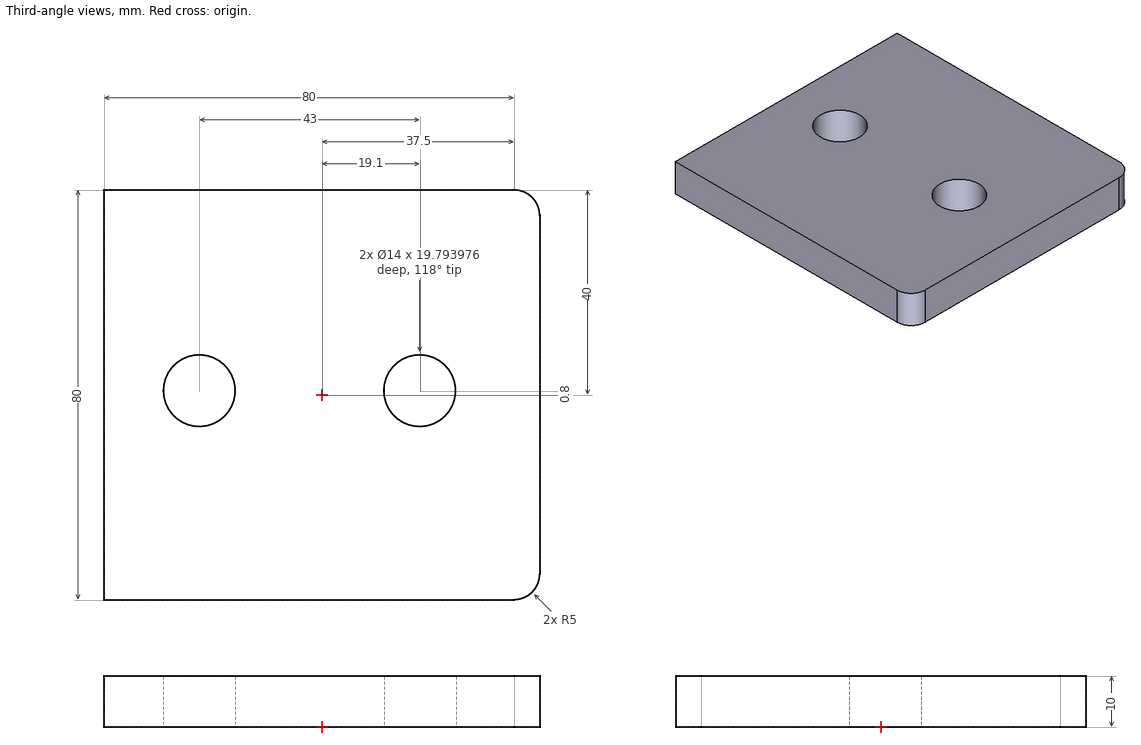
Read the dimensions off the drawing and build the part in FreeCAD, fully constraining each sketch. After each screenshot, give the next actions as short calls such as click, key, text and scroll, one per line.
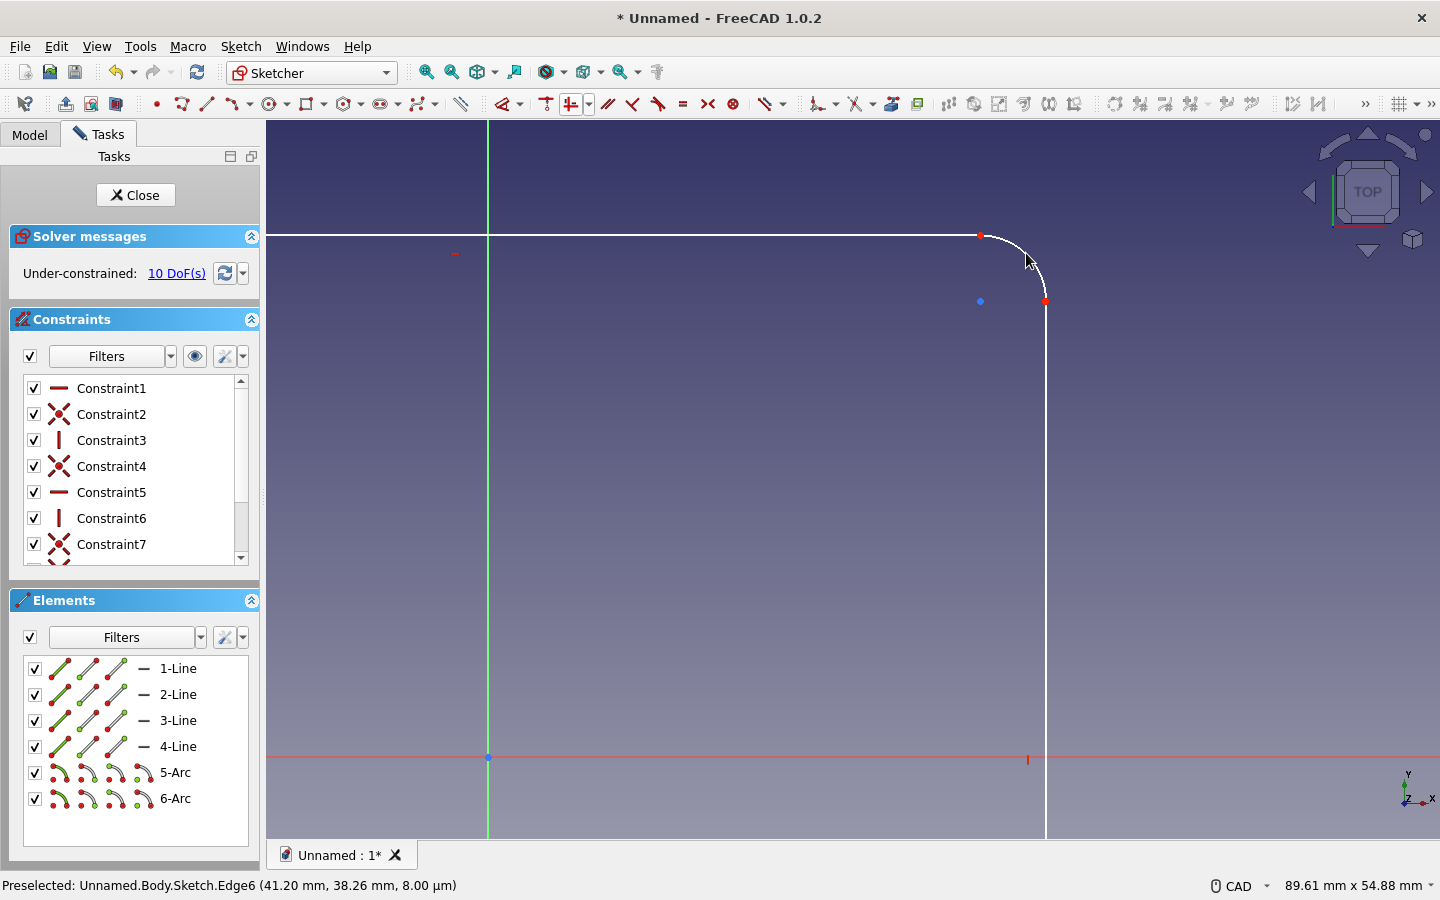
click(666, 235)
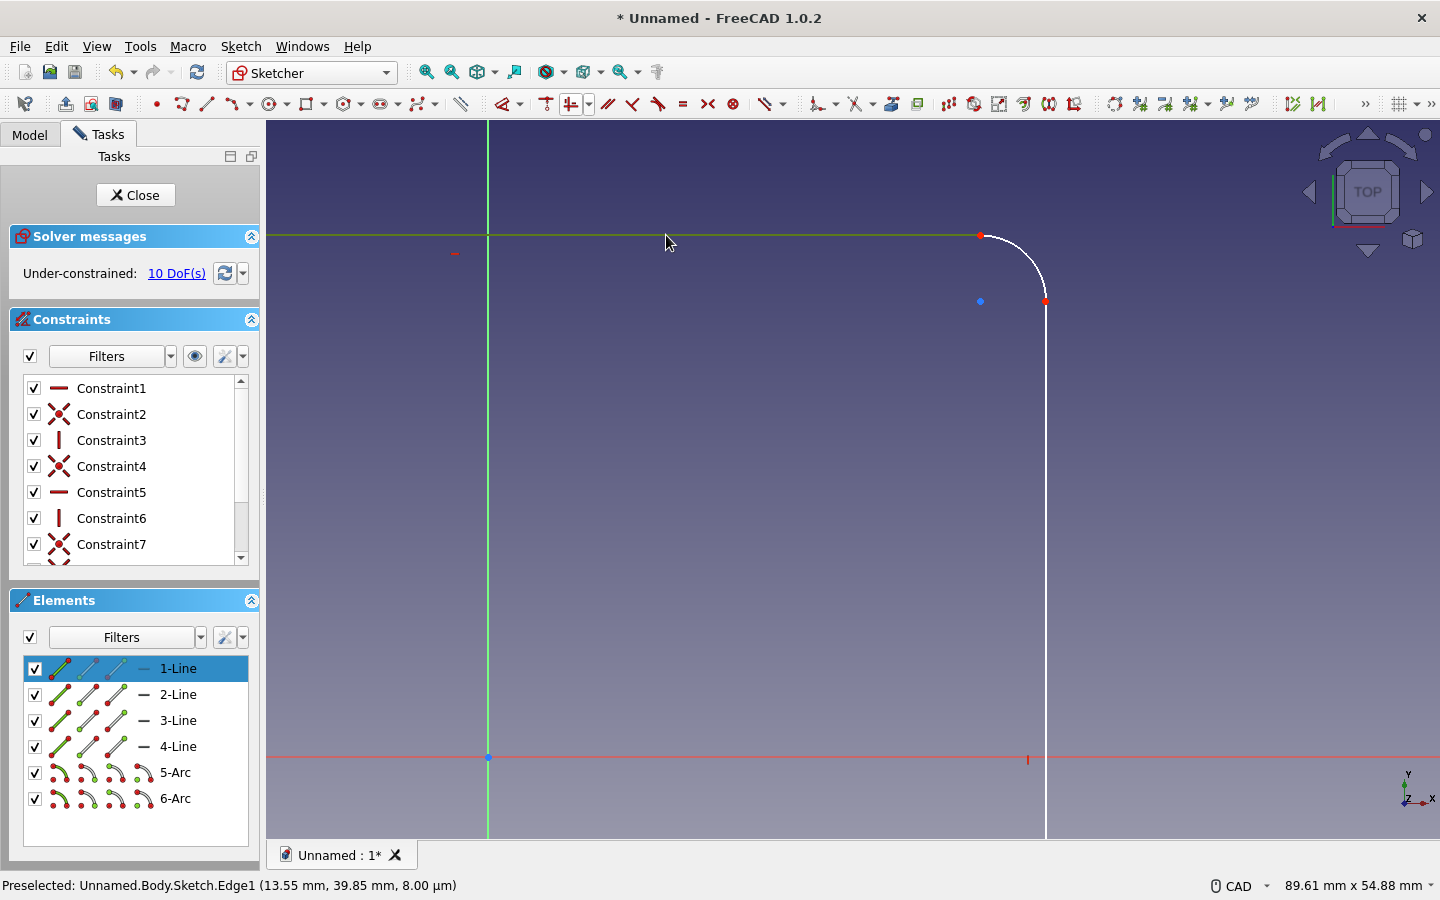
click(1039, 271)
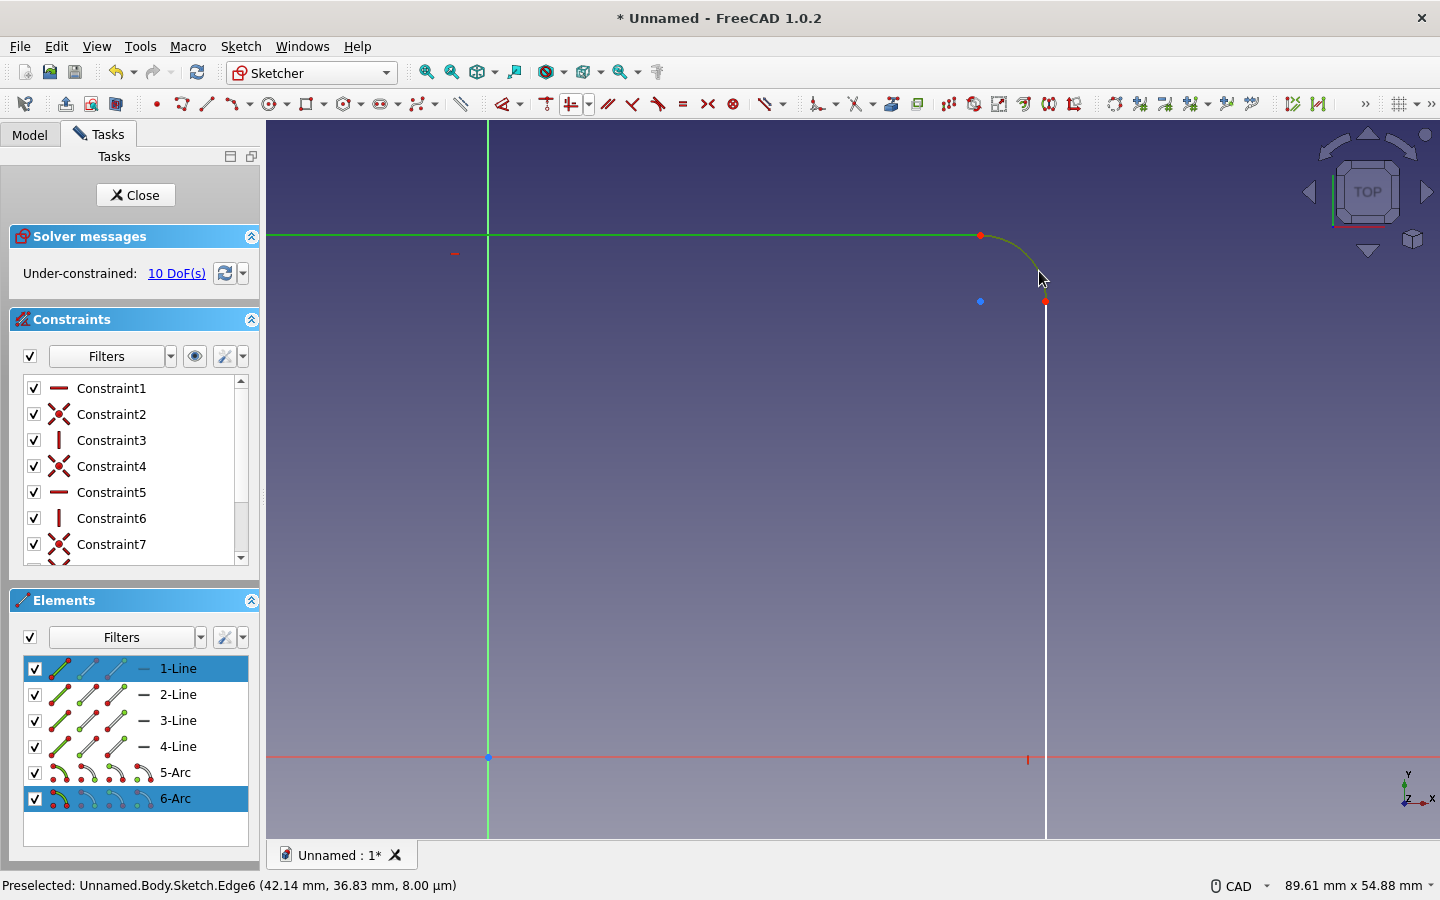
key(t)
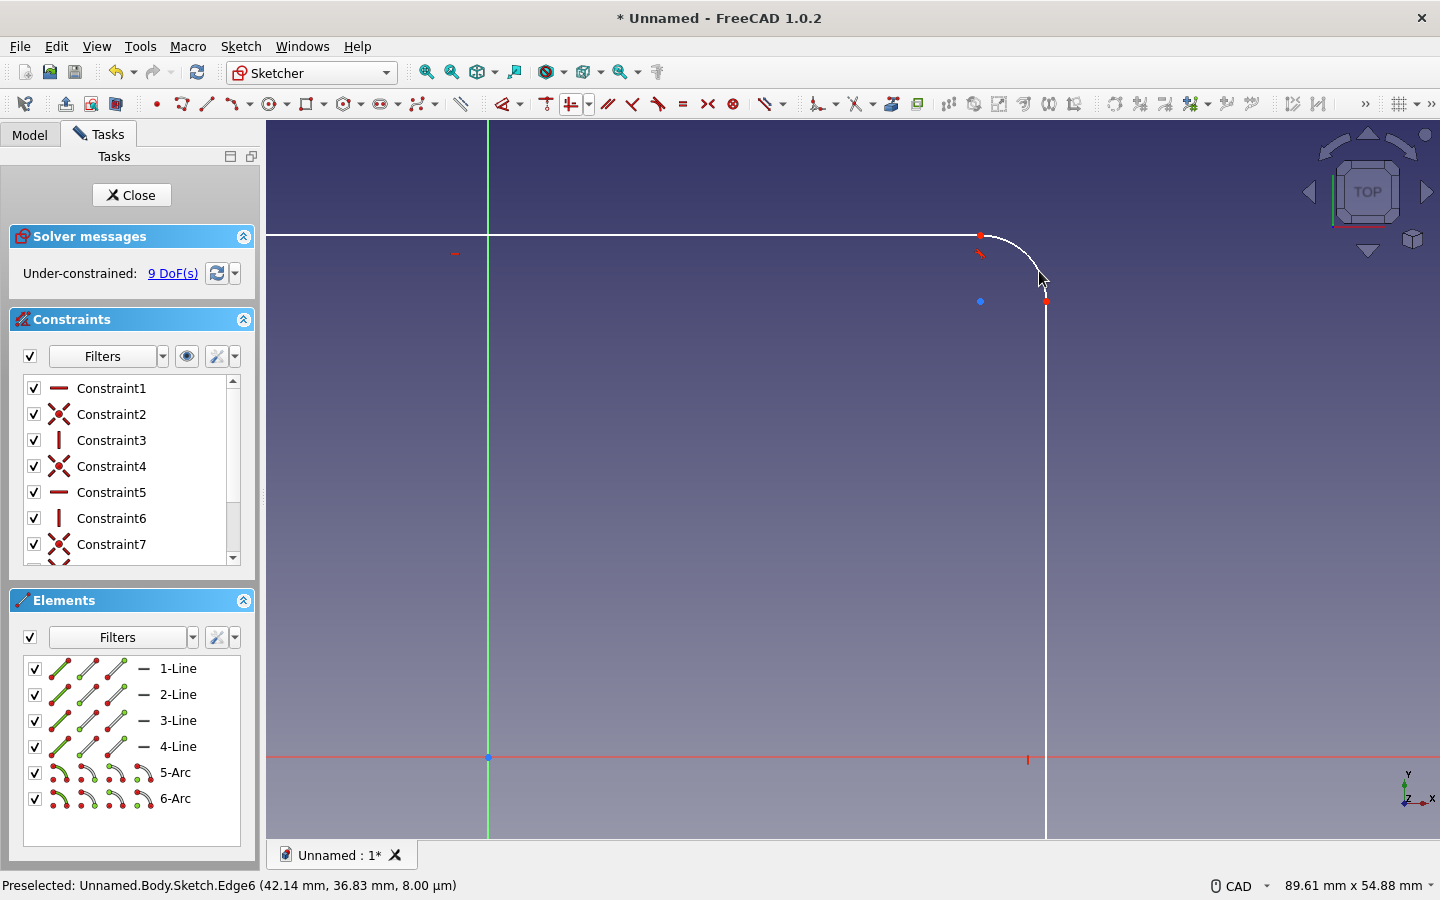
scroll(1026, 253, down, 4)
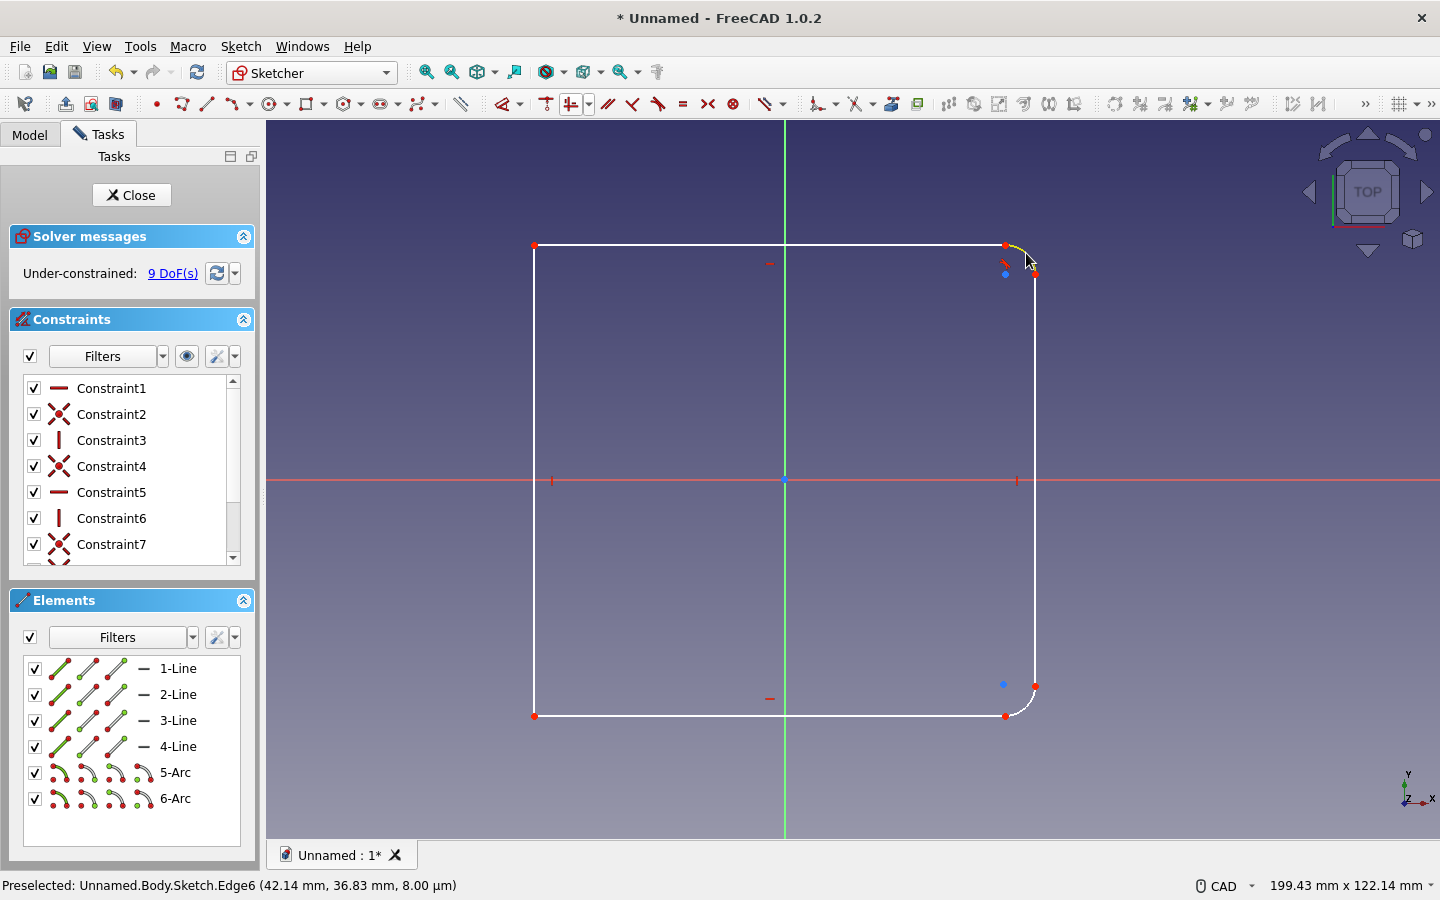
click(676, 716)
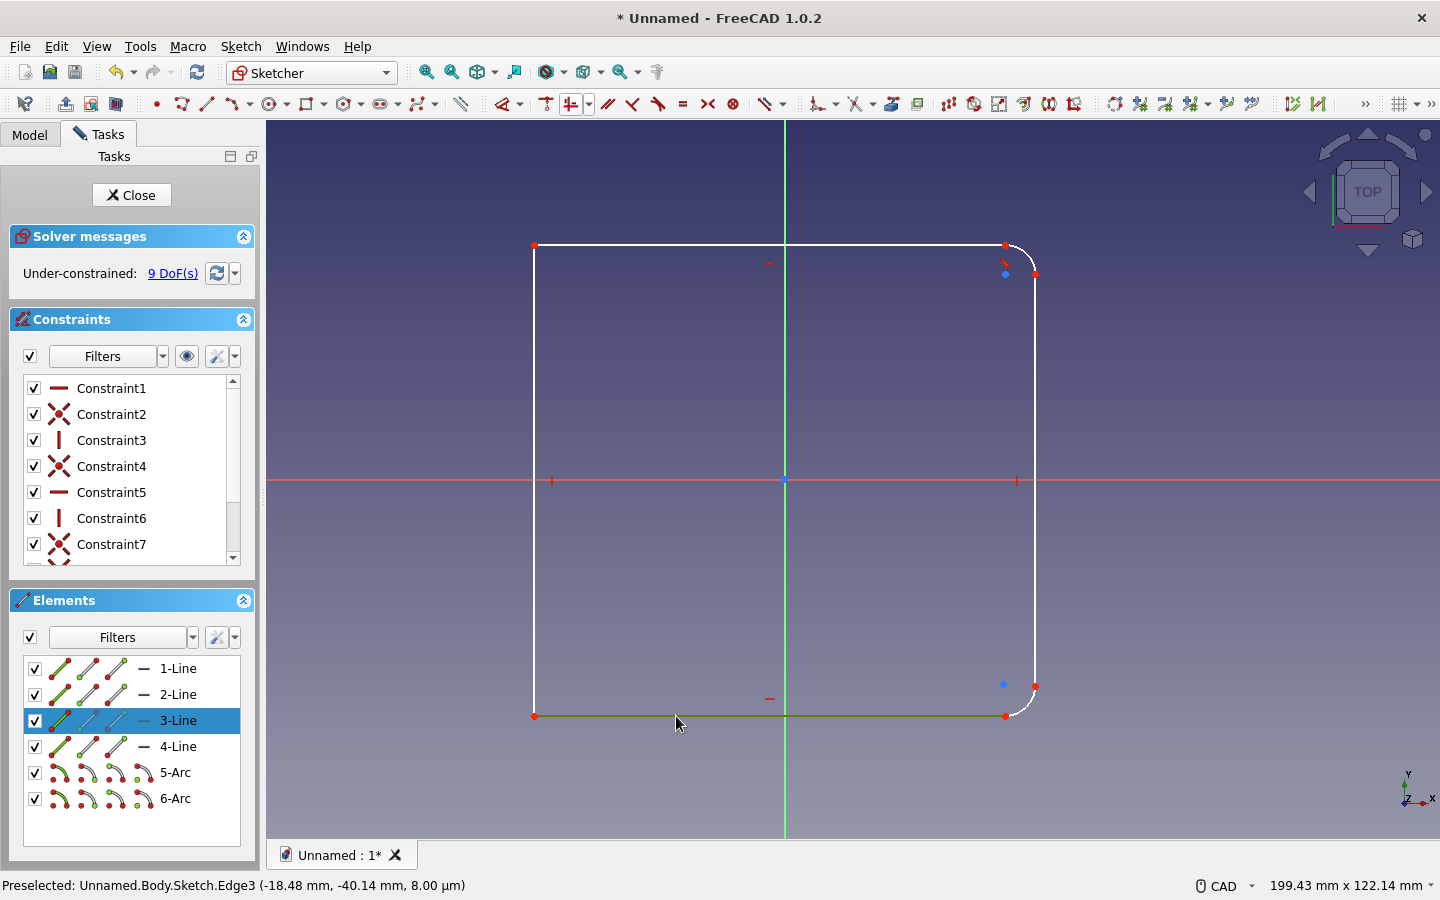
click(1019, 712)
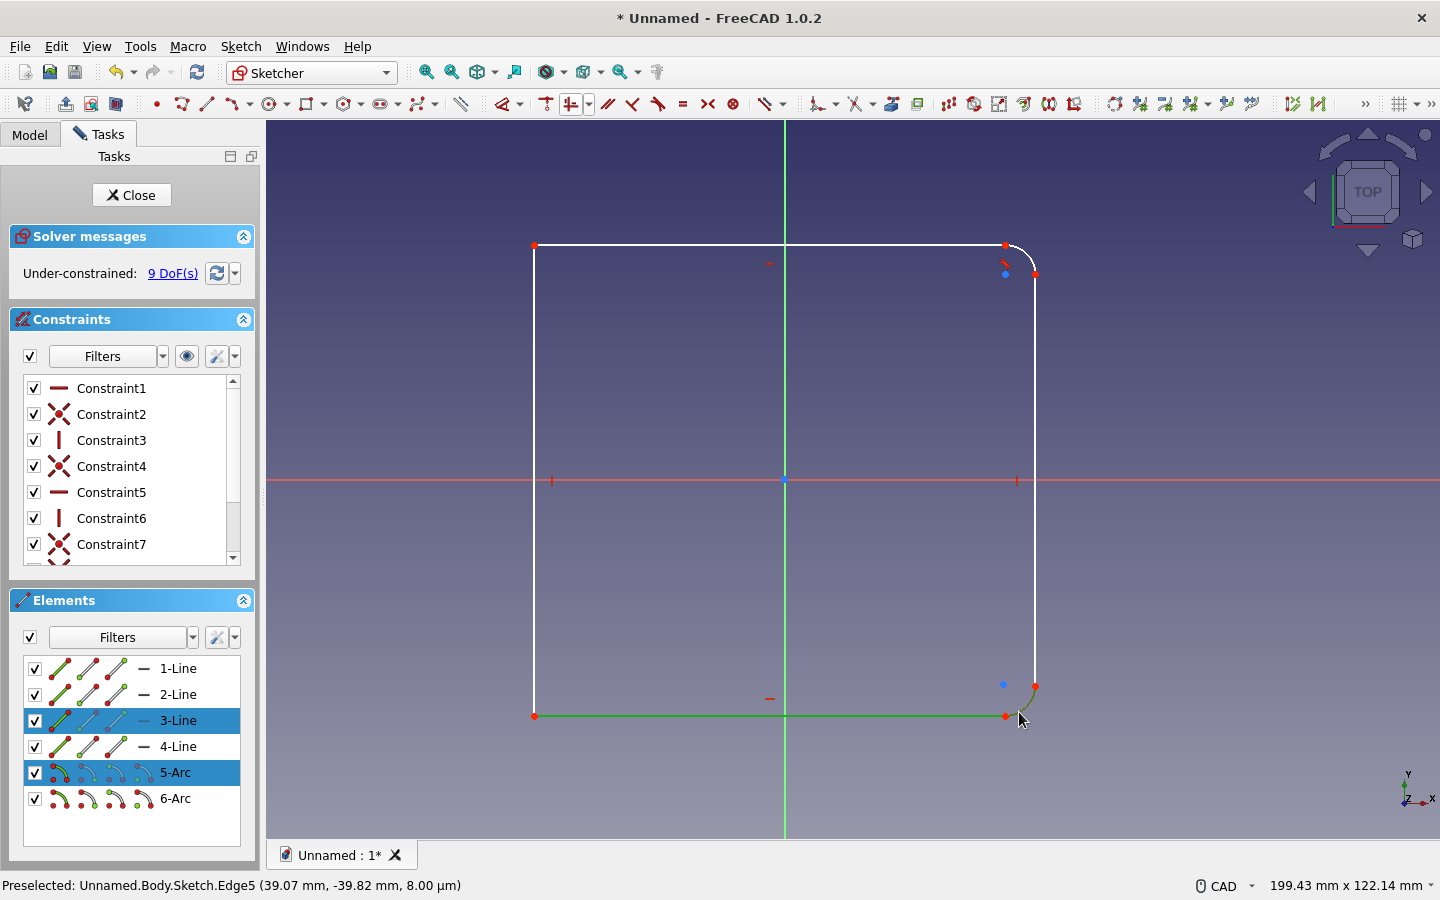
click(658, 104)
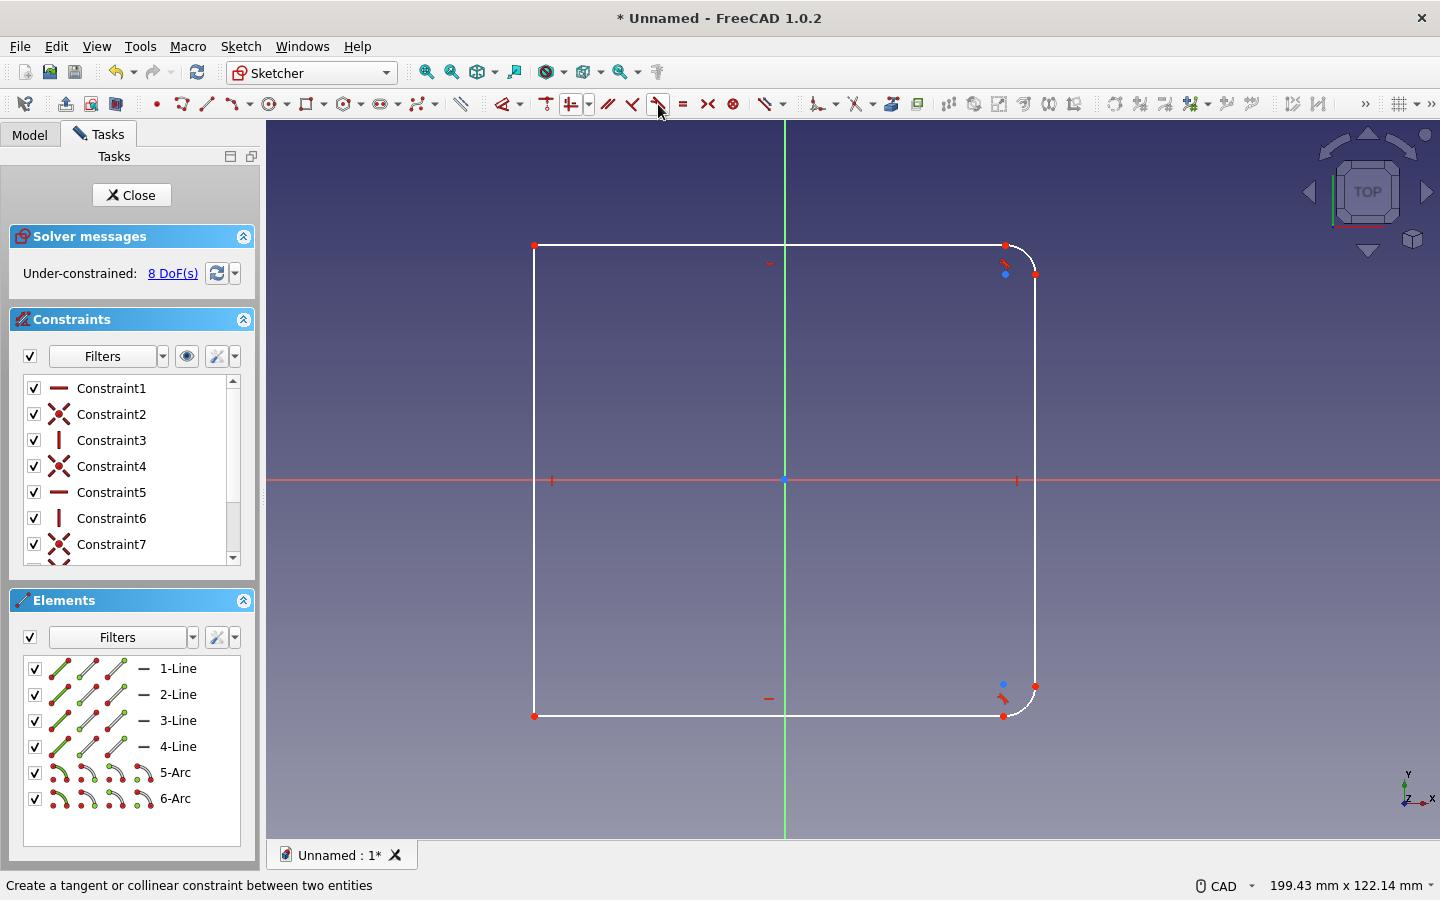
click(1035, 563)